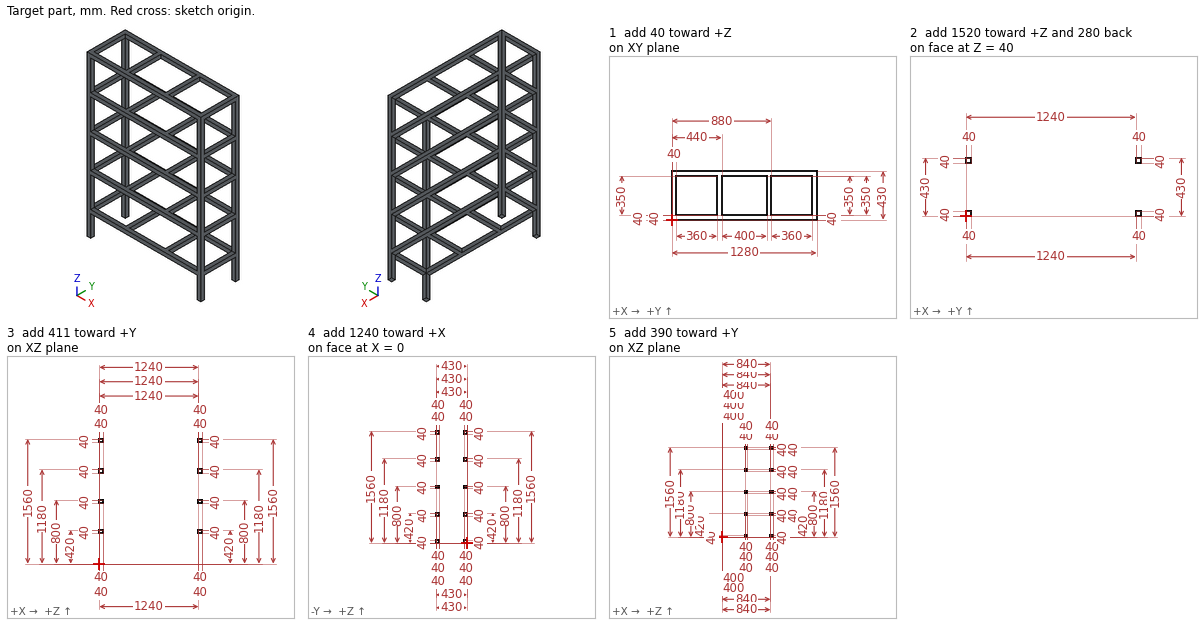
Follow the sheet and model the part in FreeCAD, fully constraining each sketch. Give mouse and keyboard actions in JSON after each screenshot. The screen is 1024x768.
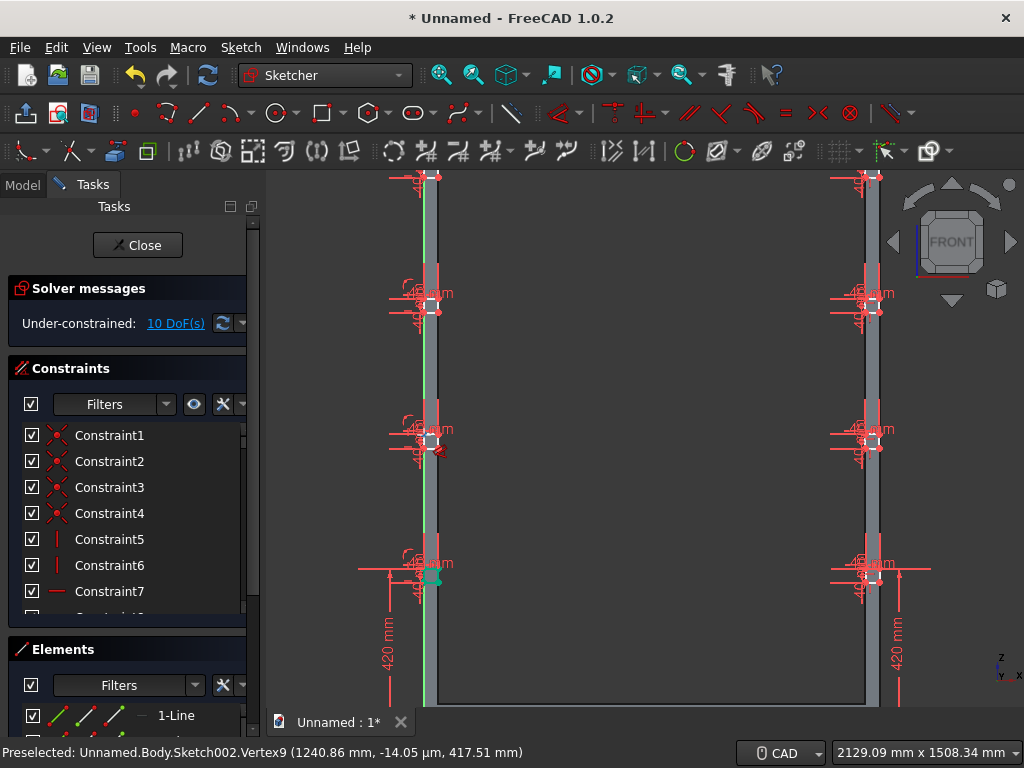
{"action": "left_click", "coordinate": [424, 434]}
{"action": "left_click", "coordinate": [390, 557]}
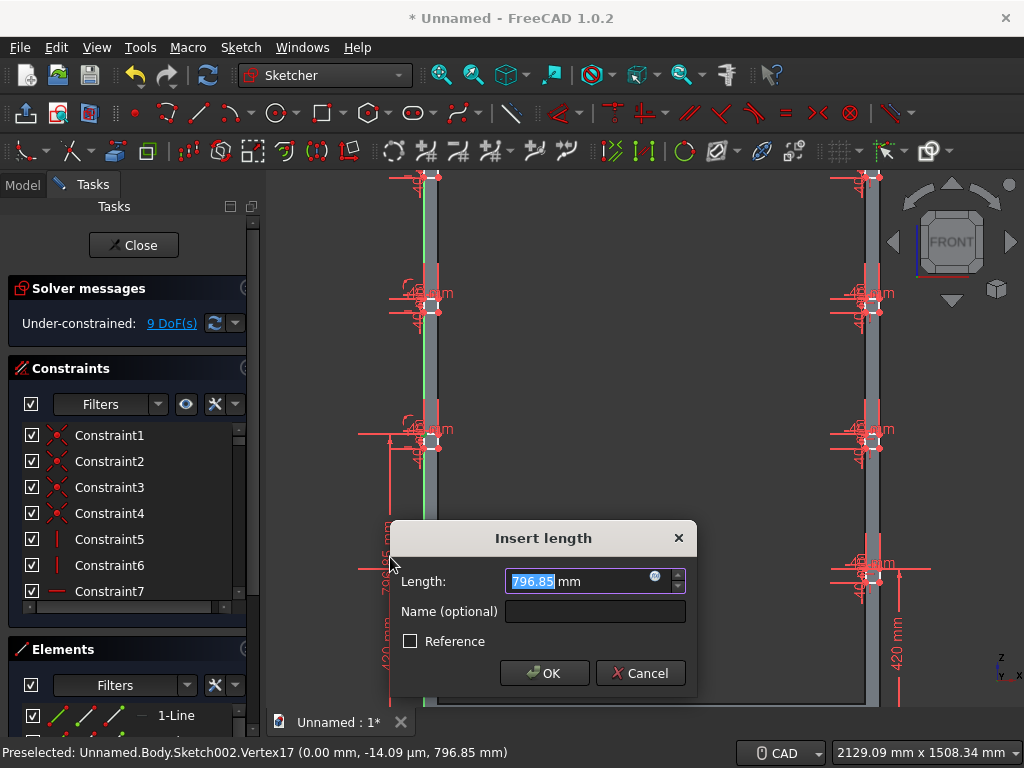
{"action": "type", "text": "800"}
{"action": "key", "text": "Return"}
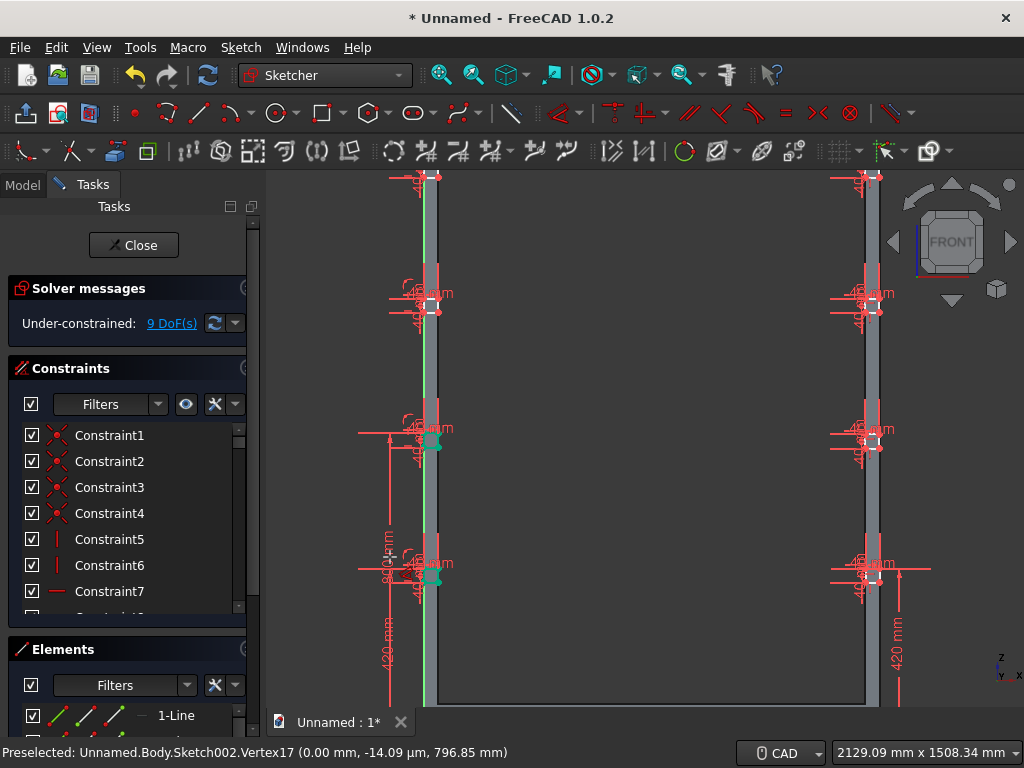
{"action": "scroll", "coordinate": [423, 435], "scroll_direction": "down", "scroll_amount": 2}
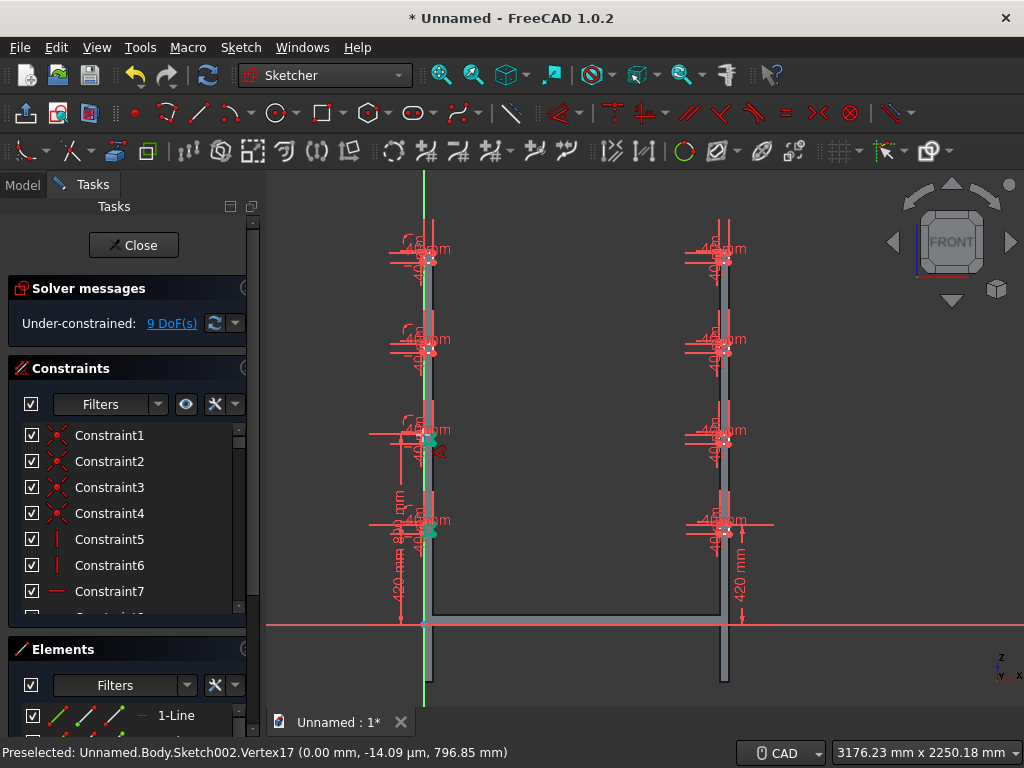
{"action": "scroll", "coordinate": [719, 435], "scroll_direction": "up", "scroll_amount": 2}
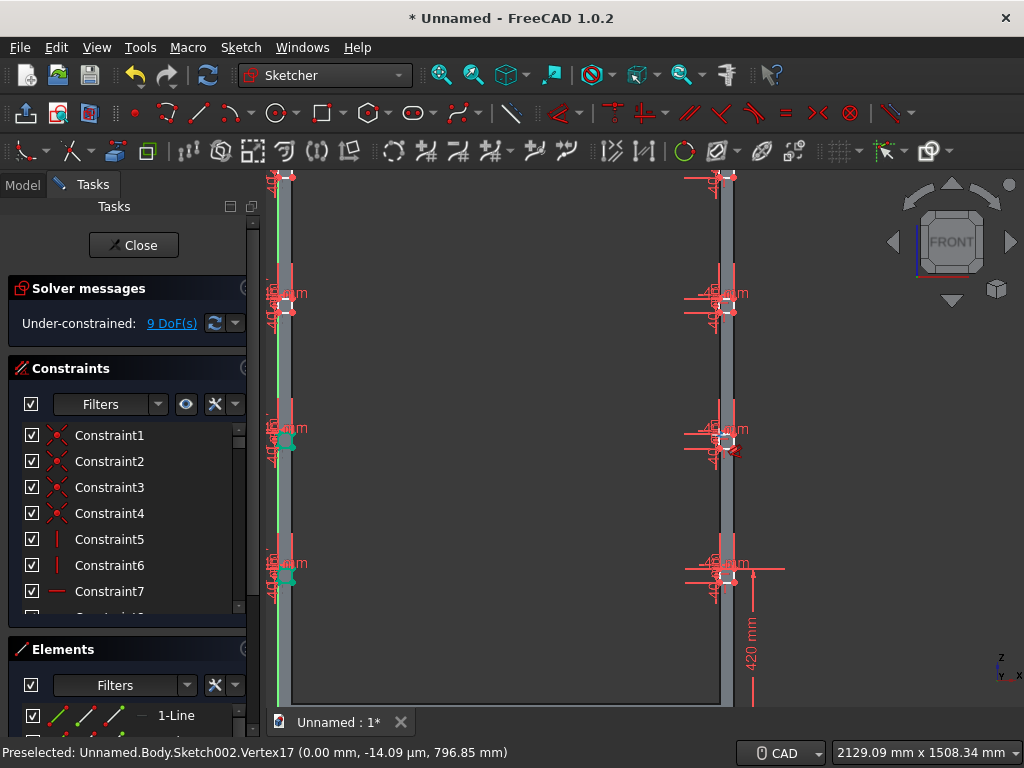
{"action": "left_click", "coordinate": [719, 434]}
{"action": "left_click", "coordinate": [753, 557]}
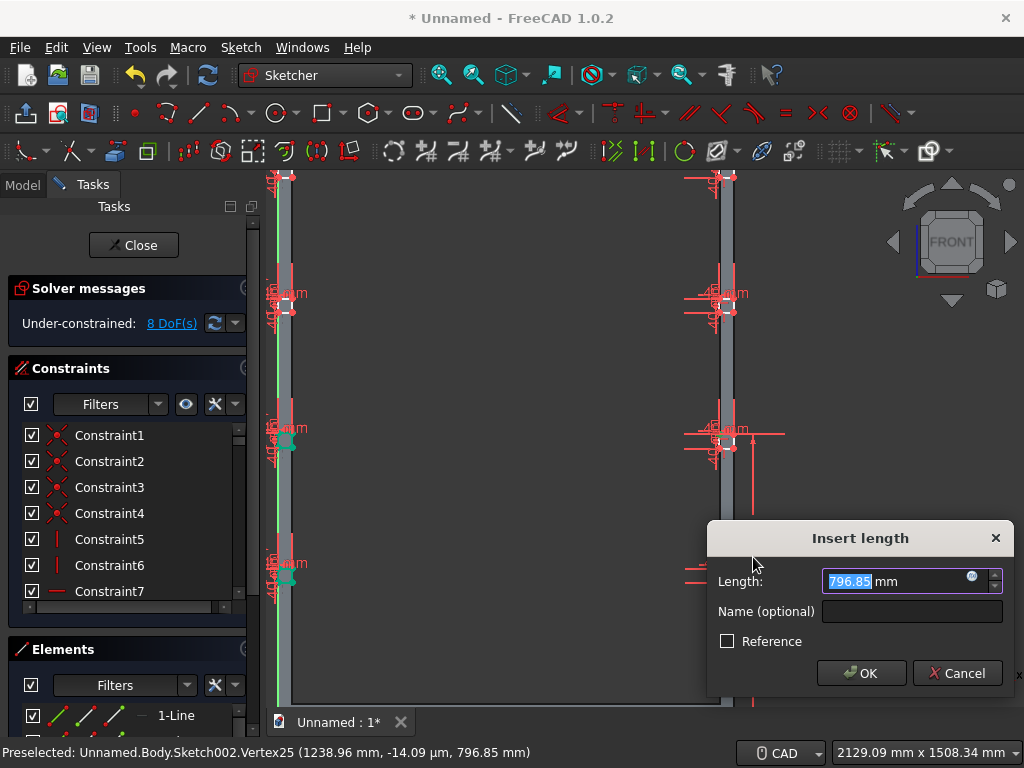
{"action": "type", "text": "800"}
{"action": "key", "text": "Return"}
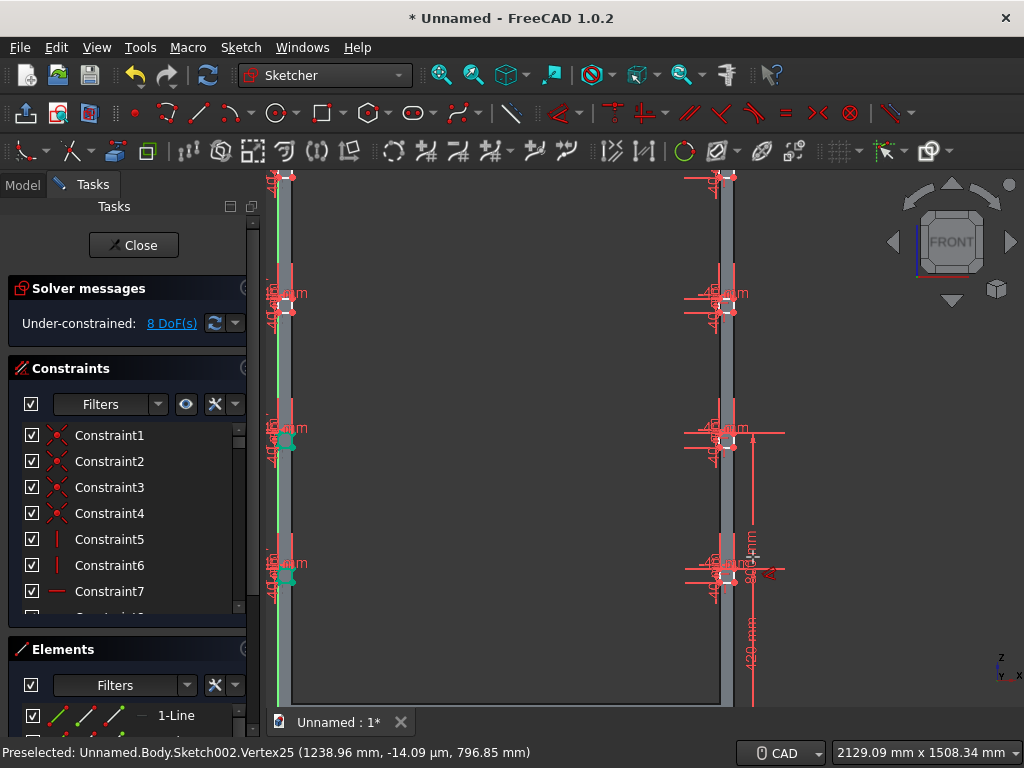
{"action": "left_click", "coordinate": [720, 569]}
{"action": "left_click", "coordinate": [507, 535]}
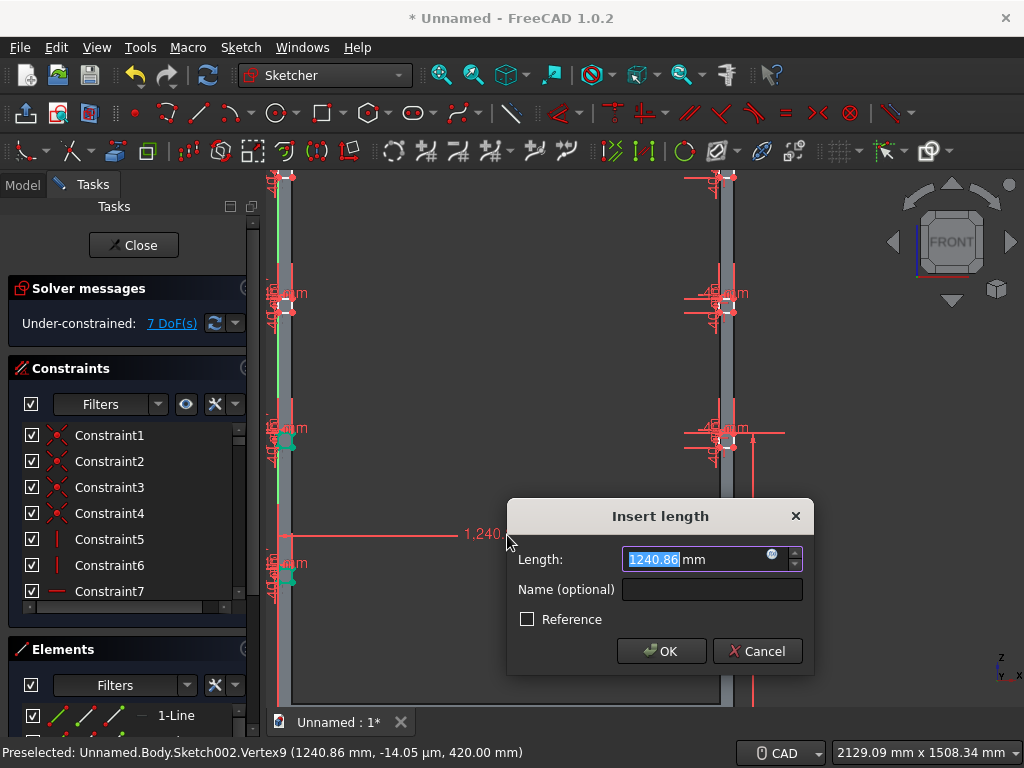
{"action": "type", "text": "1240"}
{"action": "key", "text": "Return"}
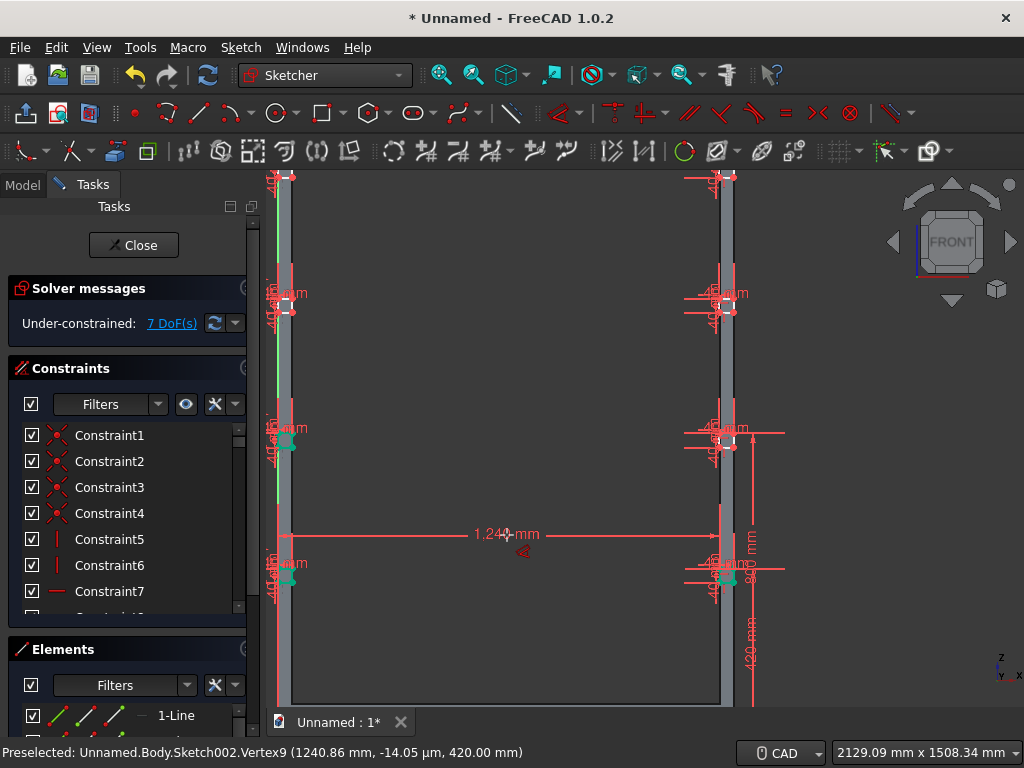
{"action": "left_click", "coordinate": [719, 433]}
{"action": "left_click", "coordinate": [507, 399]}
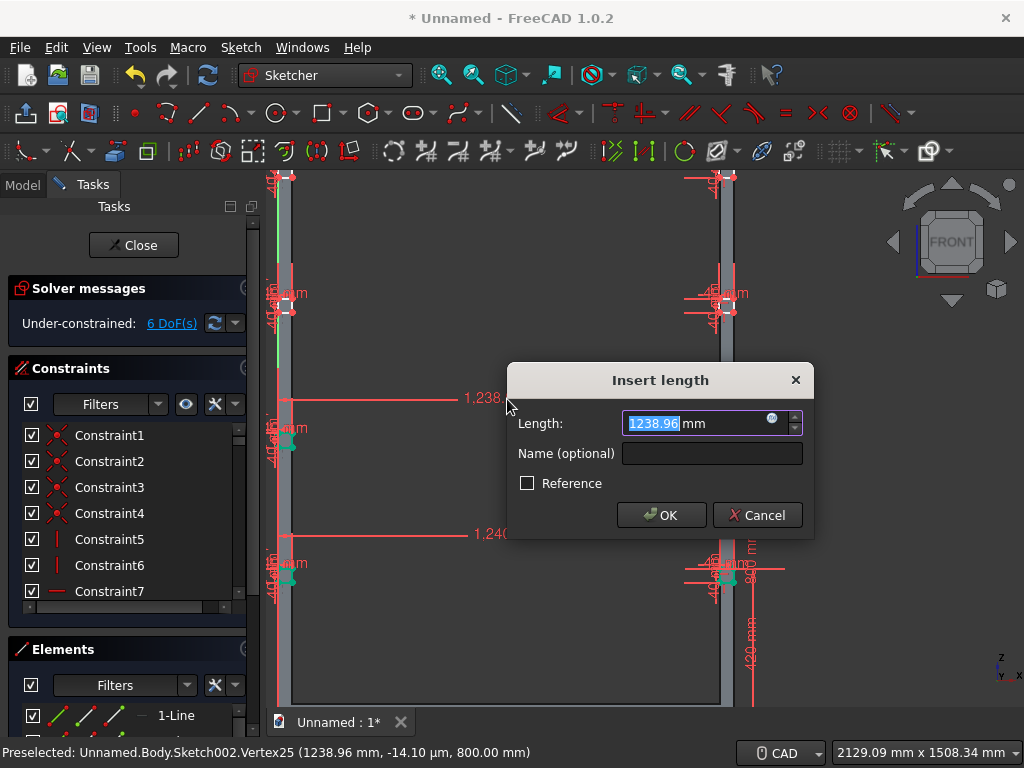
{"action": "type", "text": "1240"}
{"action": "key", "text": "Return"}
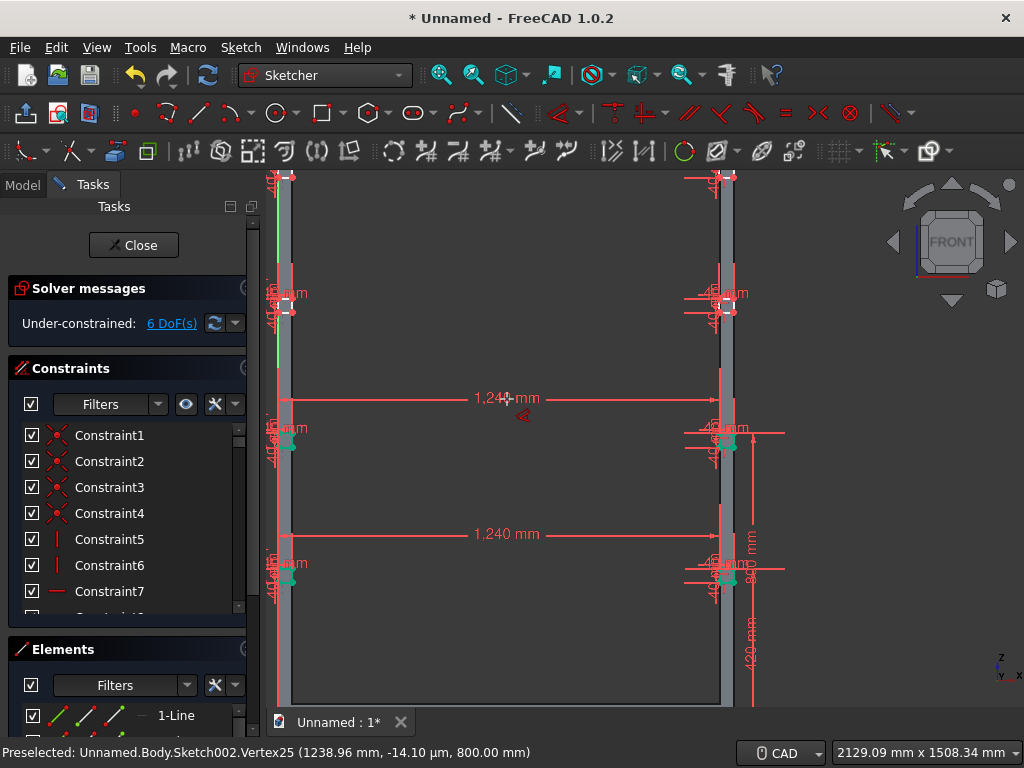
{"action": "scroll", "coordinate": [720, 435], "scroll_direction": "down", "scroll_amount": 2}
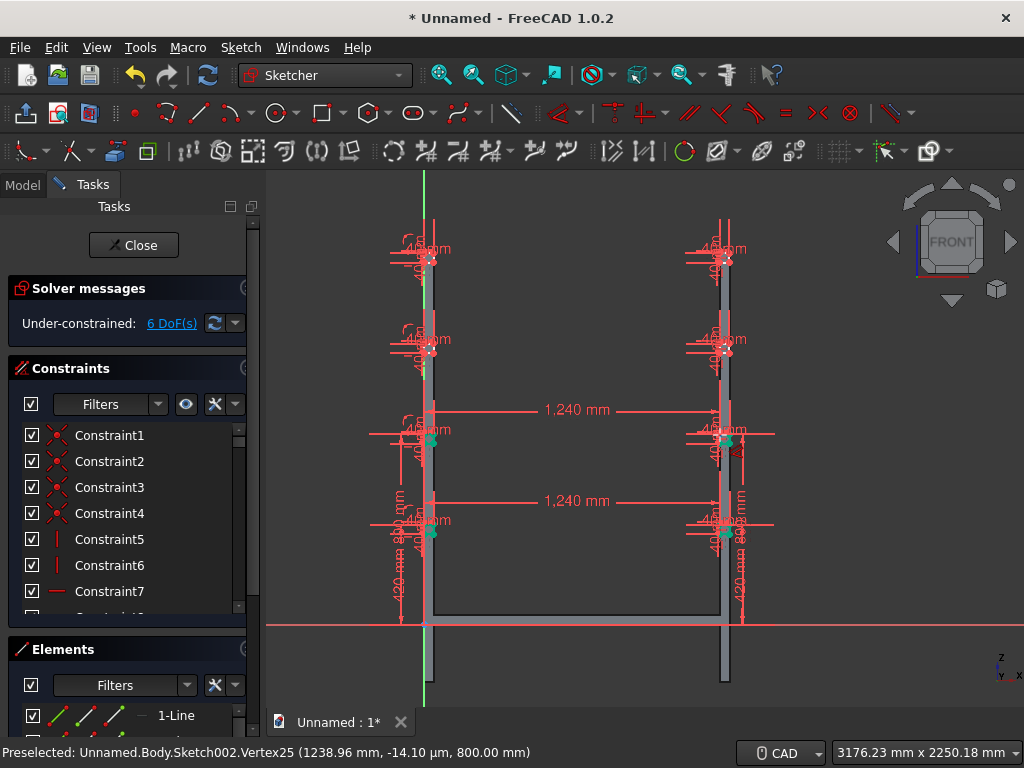
{"action": "scroll", "coordinate": [424, 344], "scroll_direction": "up", "scroll_amount": 2}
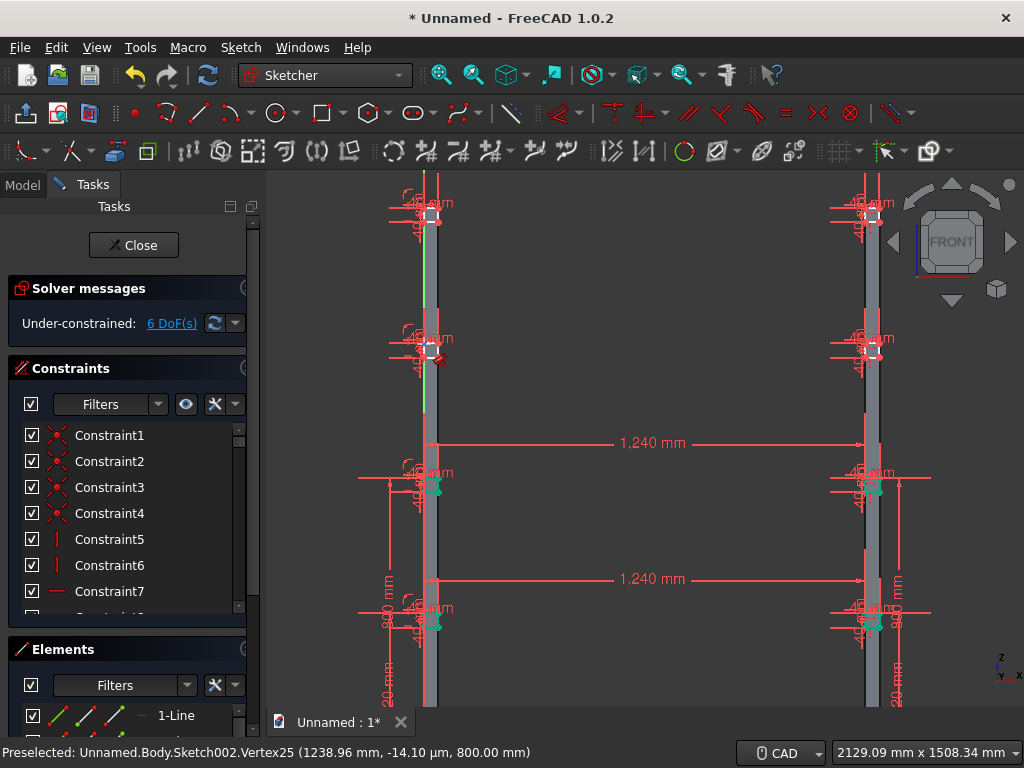
{"action": "left_click", "coordinate": [424, 343]}
{"action": "left_click", "coordinate": [390, 511]}